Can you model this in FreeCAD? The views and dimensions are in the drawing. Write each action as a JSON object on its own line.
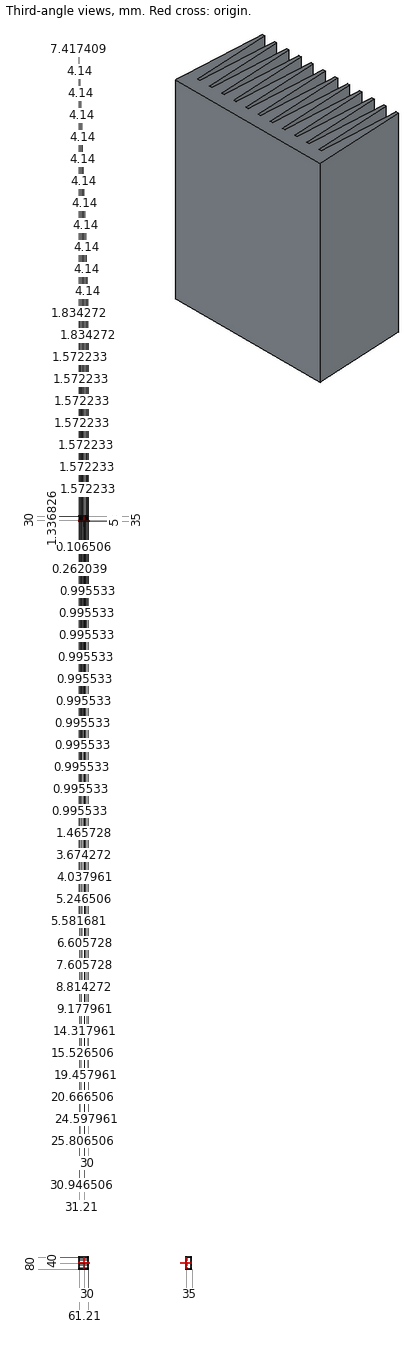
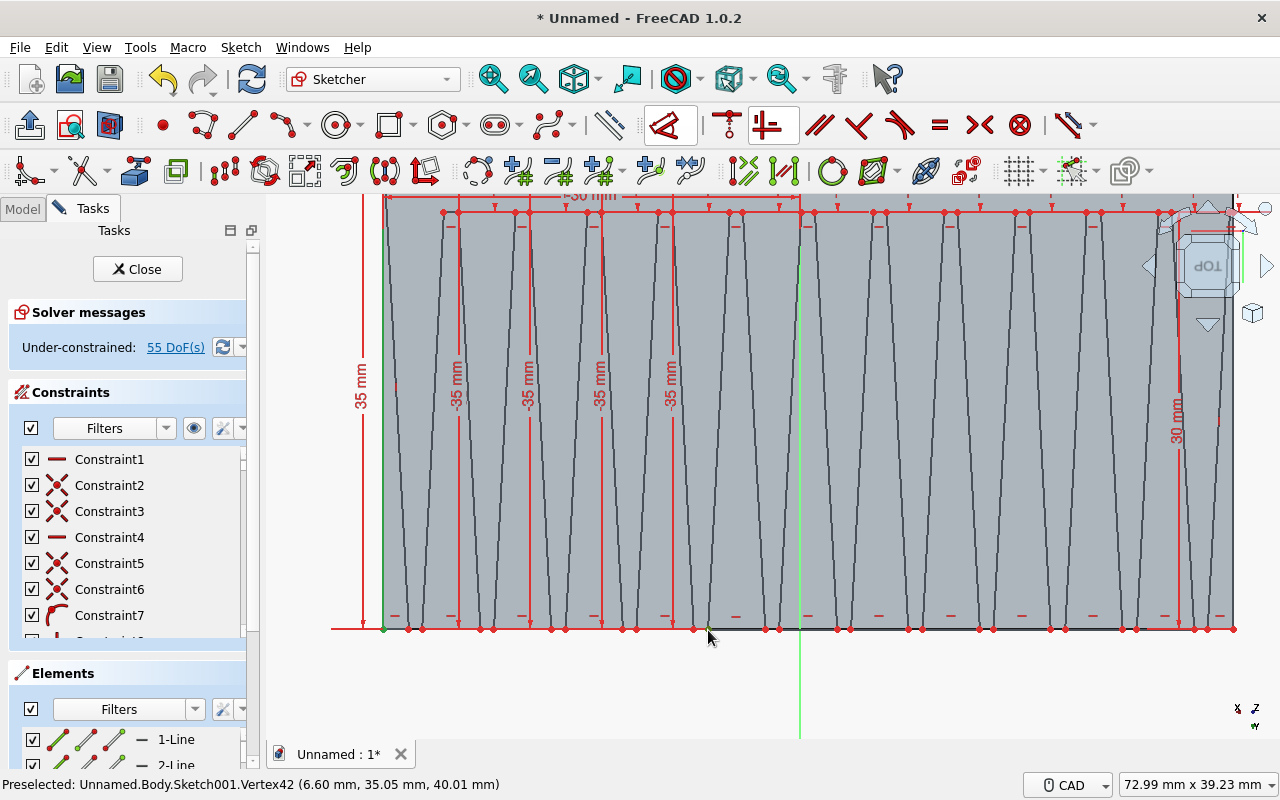
{"action": "left_click", "coordinate": [692, 126]}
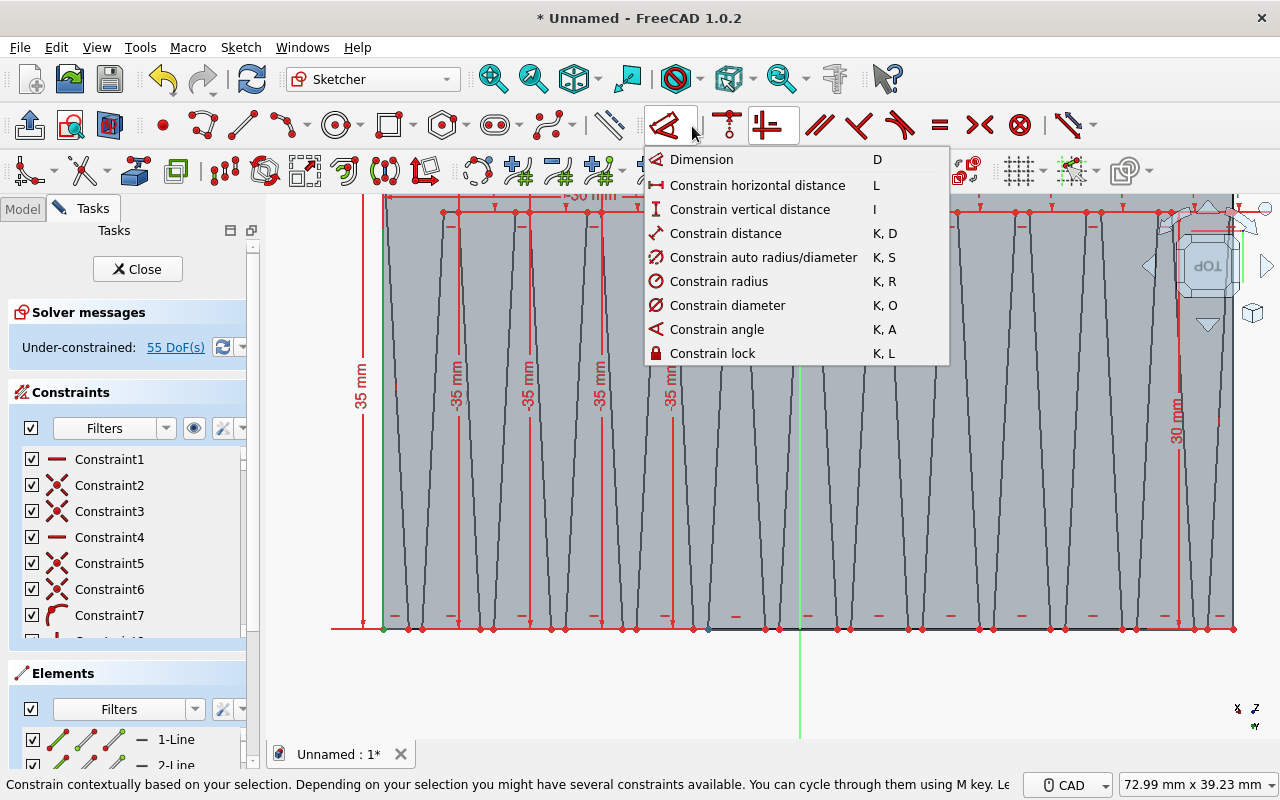
{"action": "left_click", "coordinate": [797, 209]}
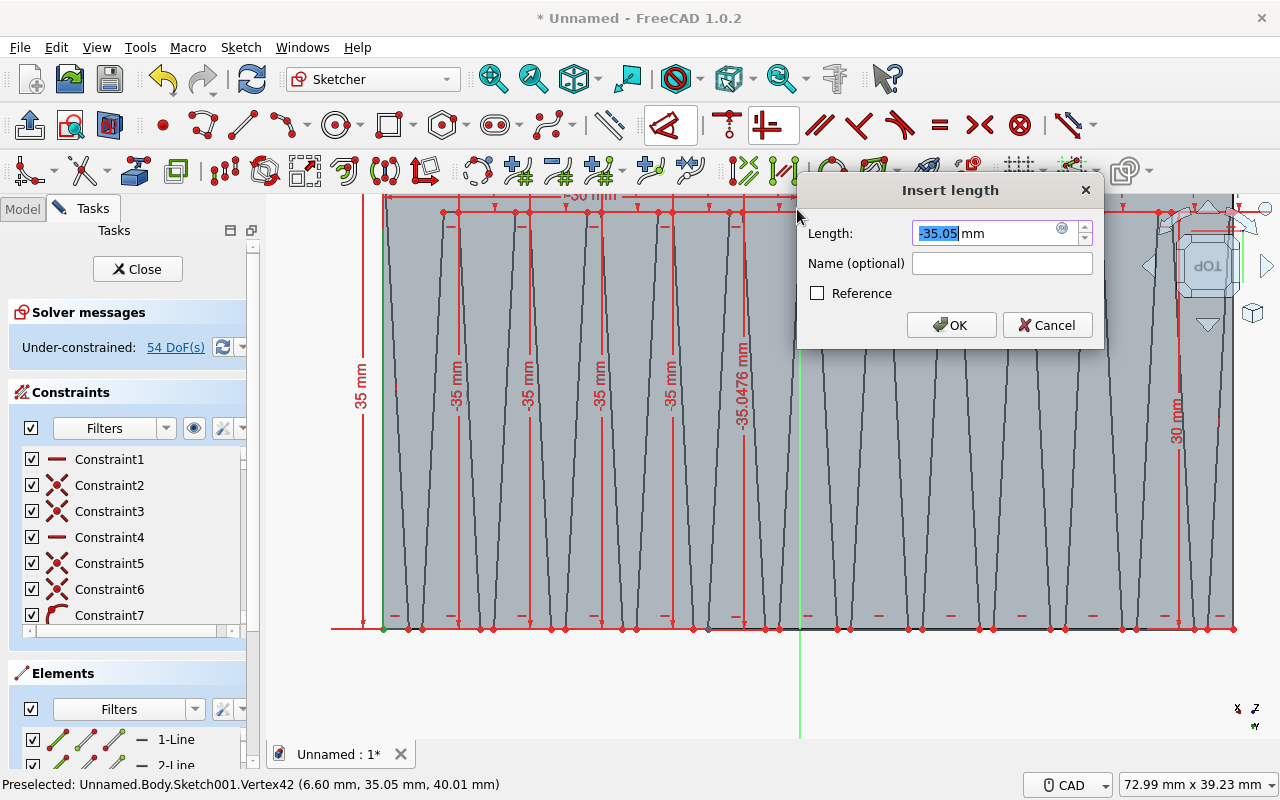
{"action": "type", "text": "-35"}
{"action": "key", "text": "Return"}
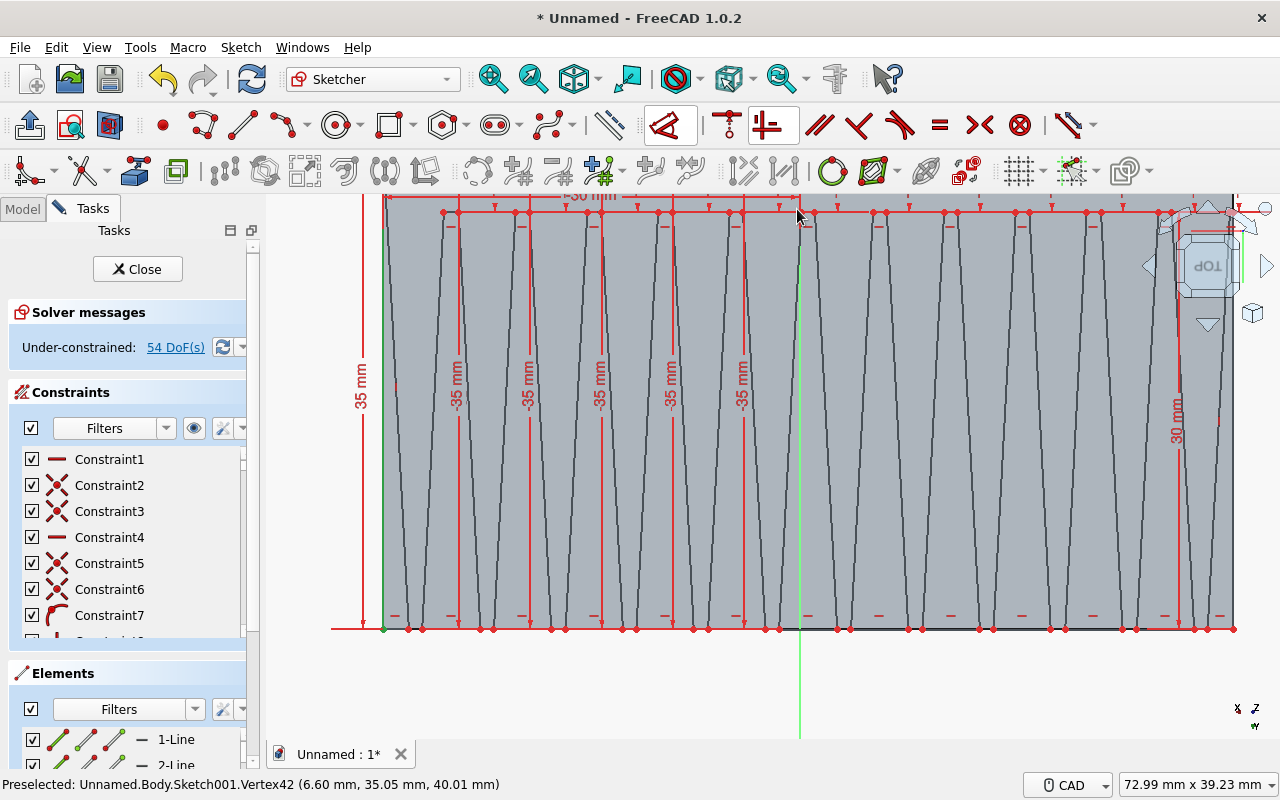
{"action": "left_click", "coordinate": [779, 630]}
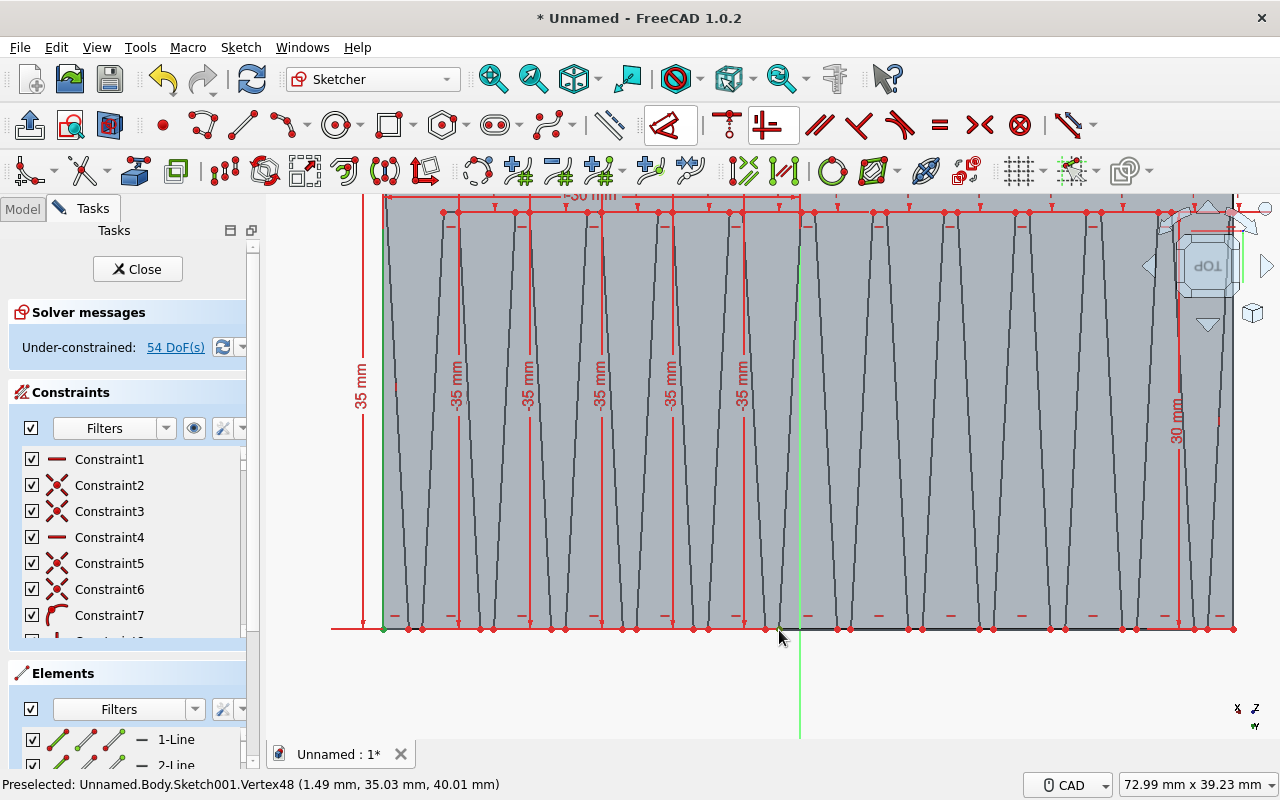
{"action": "key", "text": "i"}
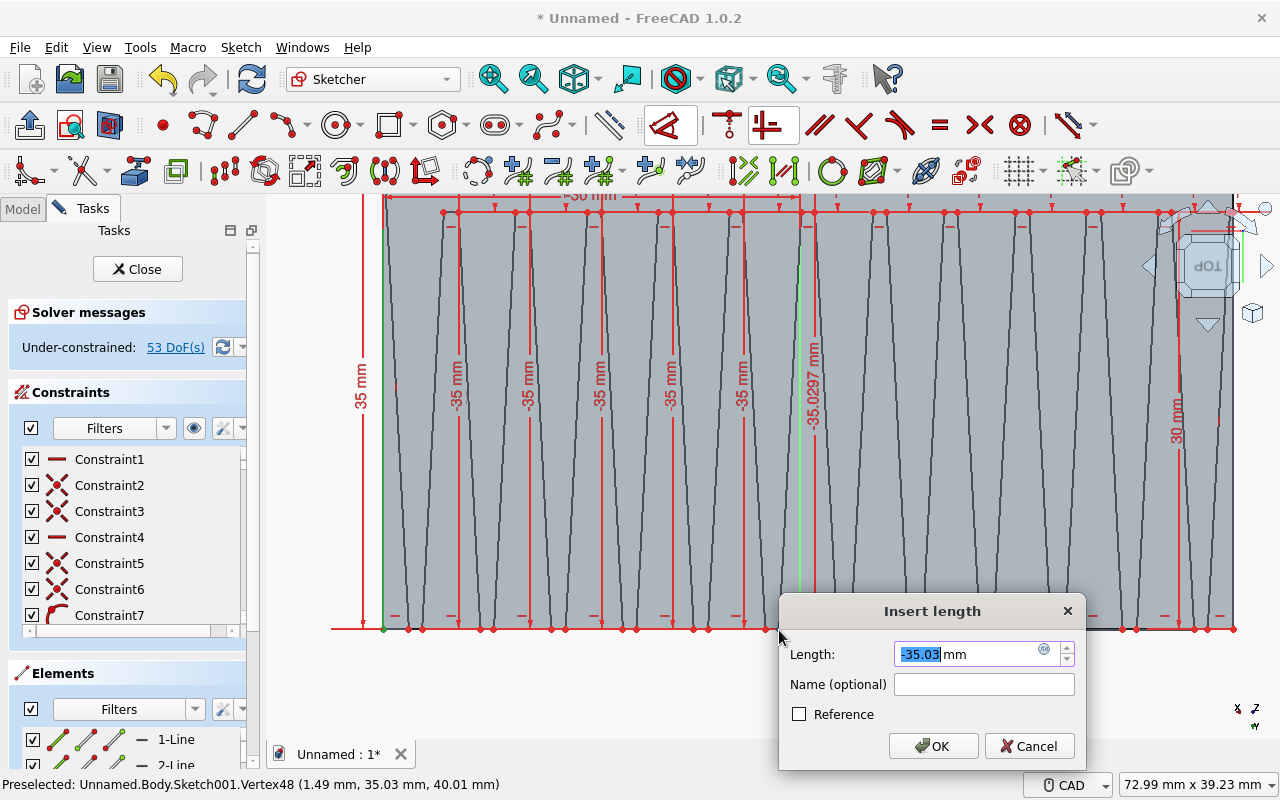
{"action": "type", "text": "-35"}
{"action": "key", "text": "Return"}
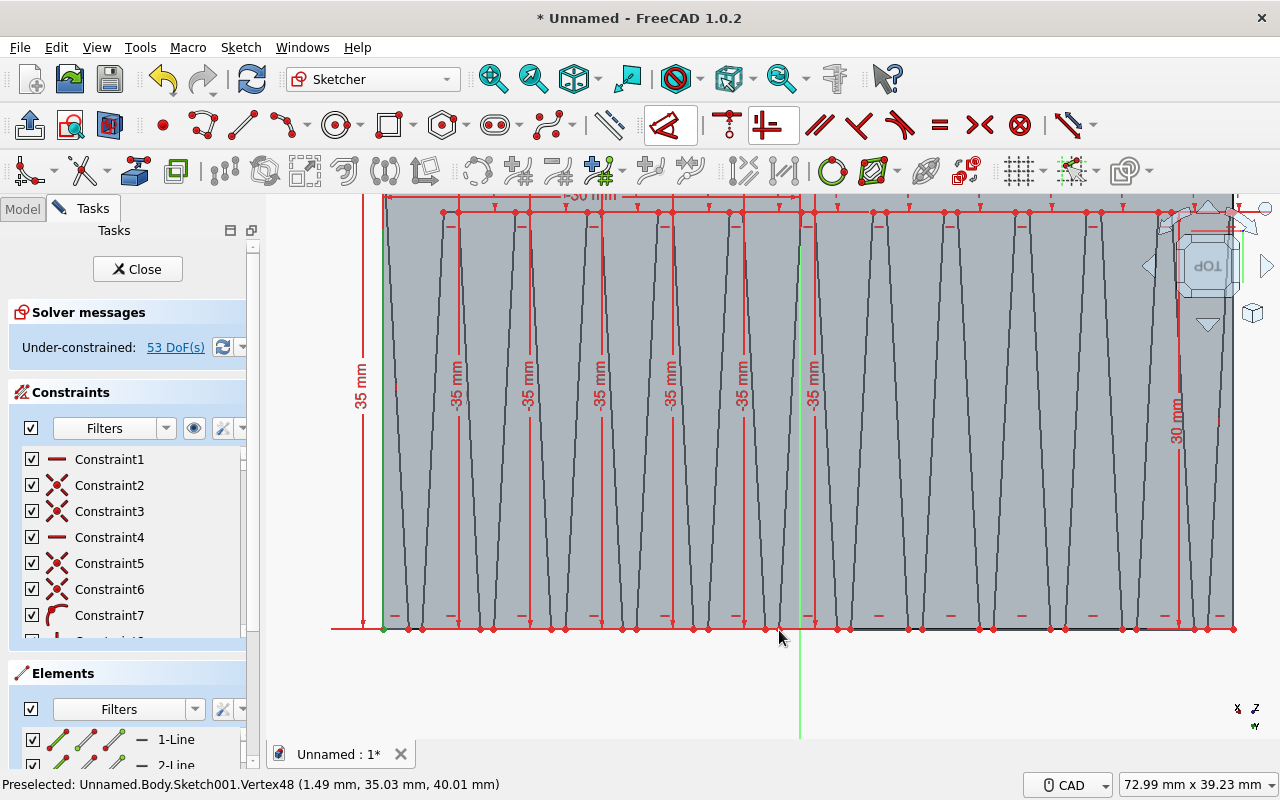
{"action": "left_click", "coordinate": [851, 630]}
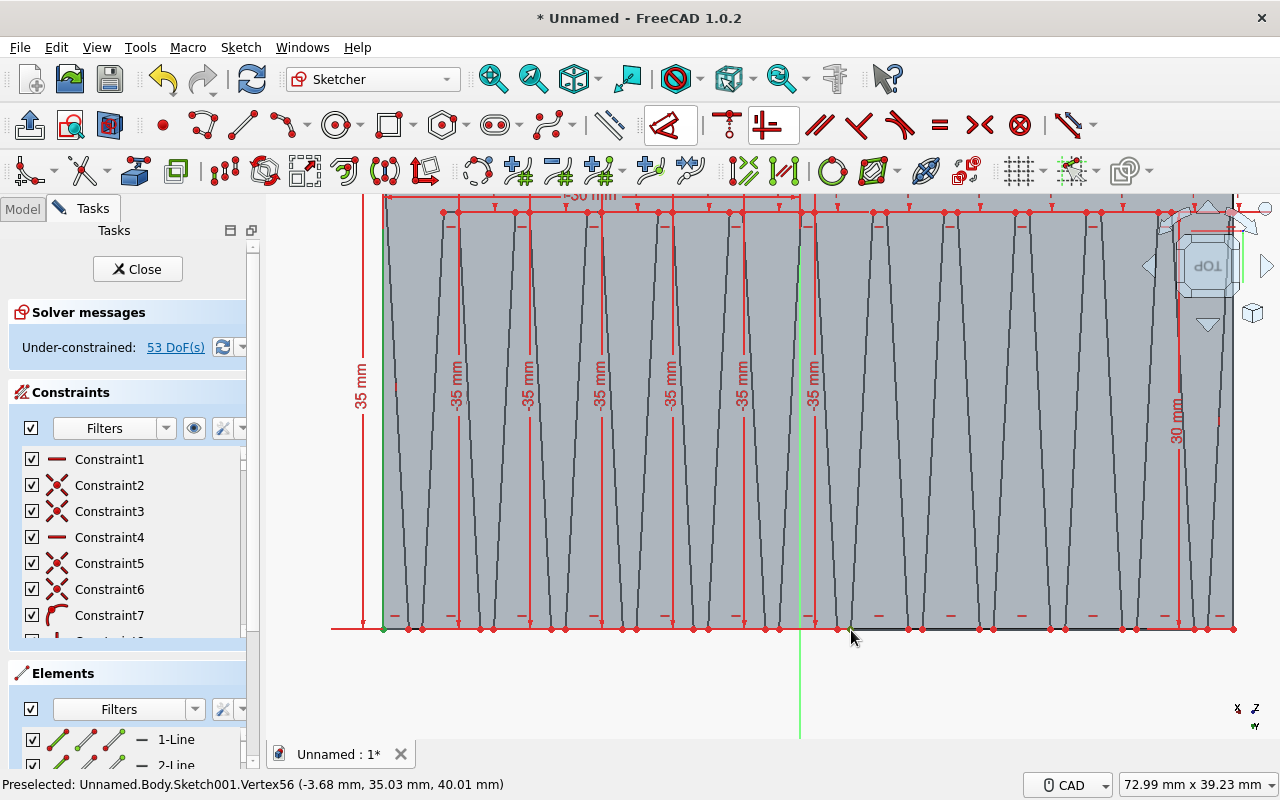
{"action": "key", "text": "i"}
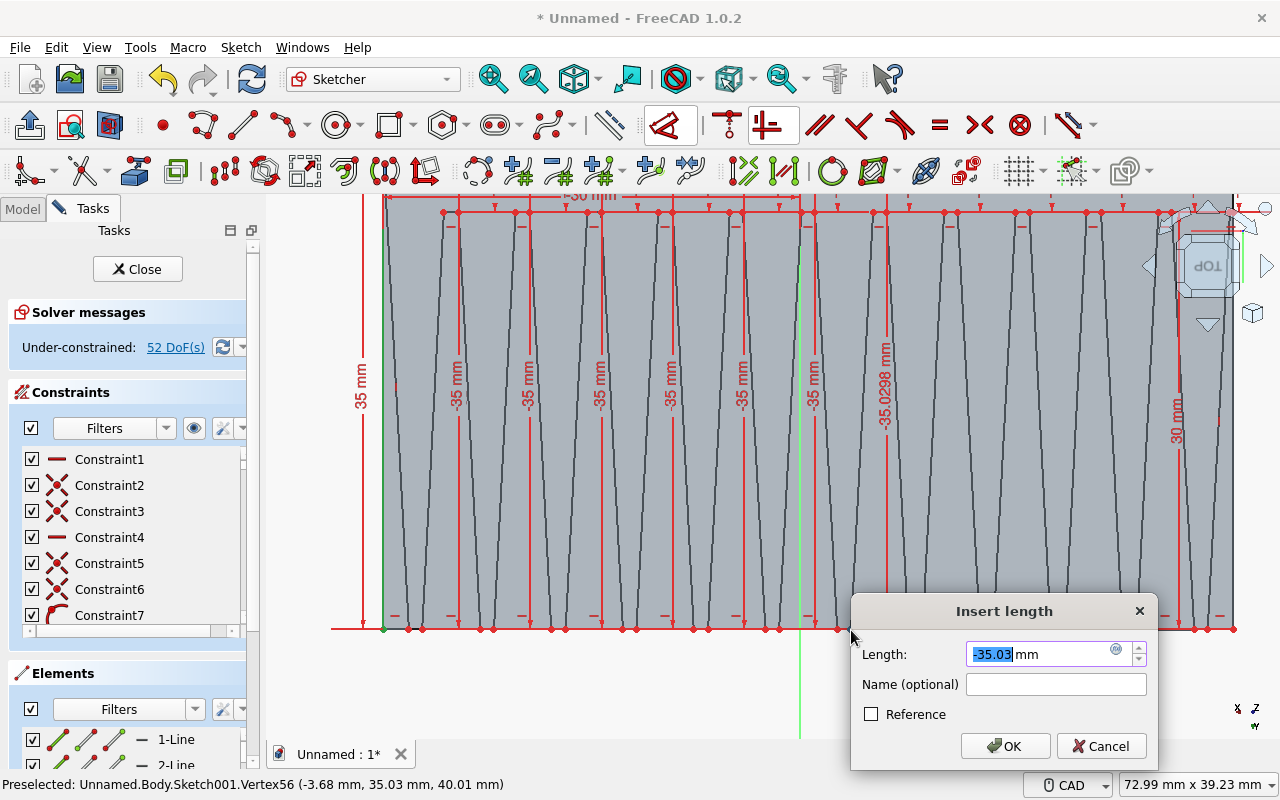
{"action": "type", "text": "-35"}
{"action": "key", "text": "Return"}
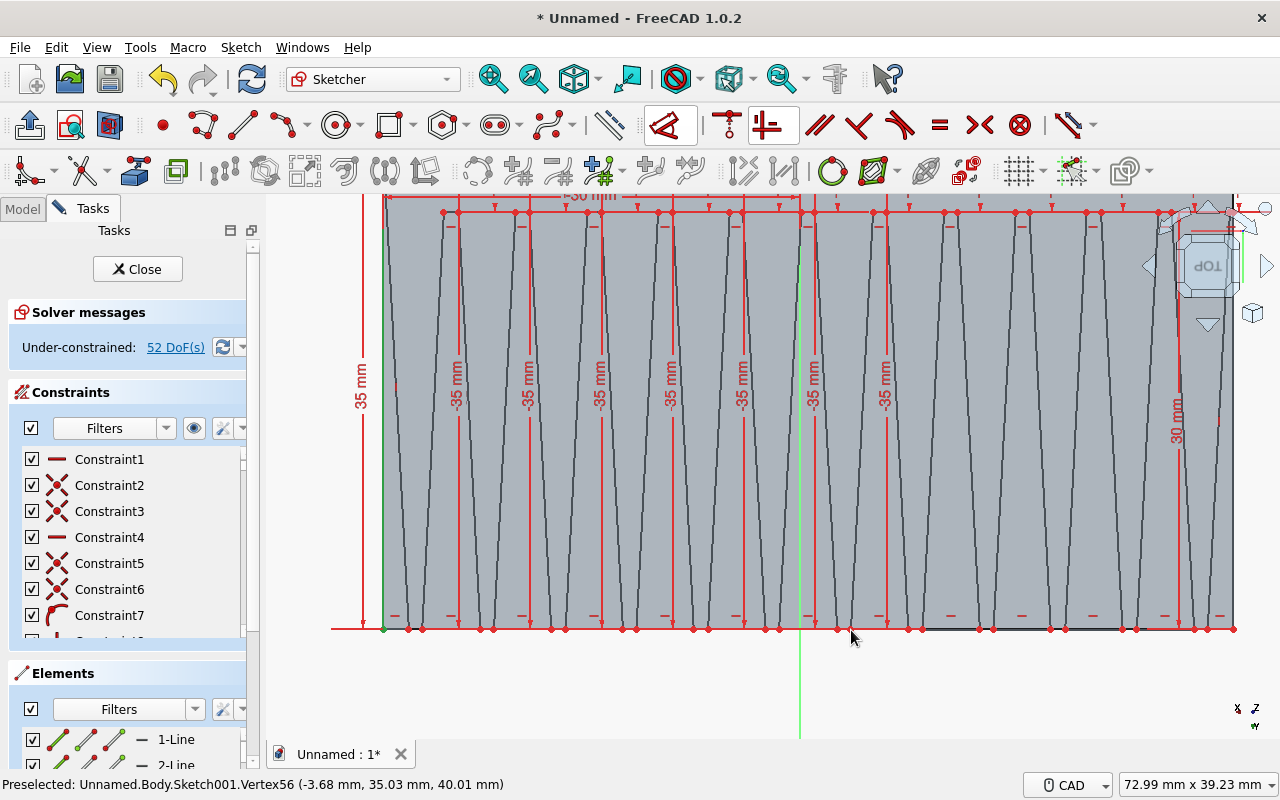
{"action": "left_click", "coordinate": [923, 630]}